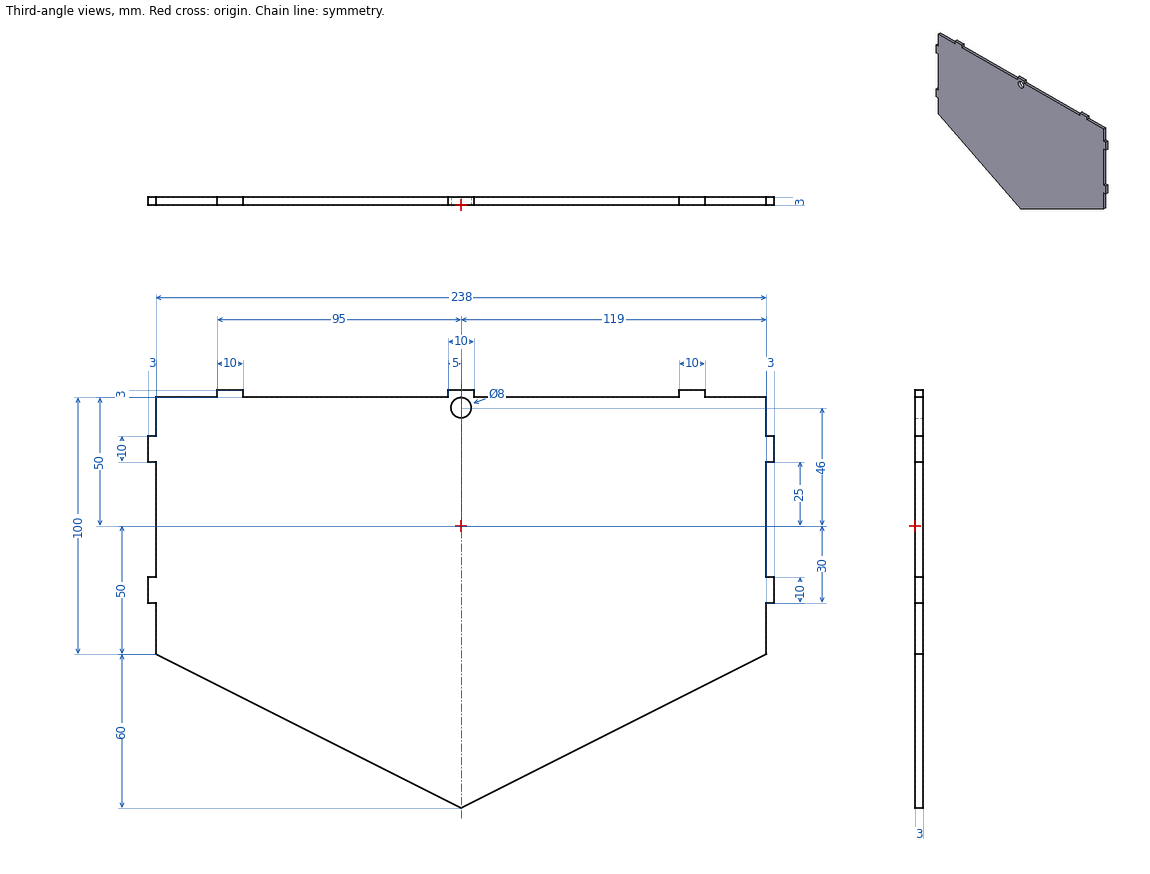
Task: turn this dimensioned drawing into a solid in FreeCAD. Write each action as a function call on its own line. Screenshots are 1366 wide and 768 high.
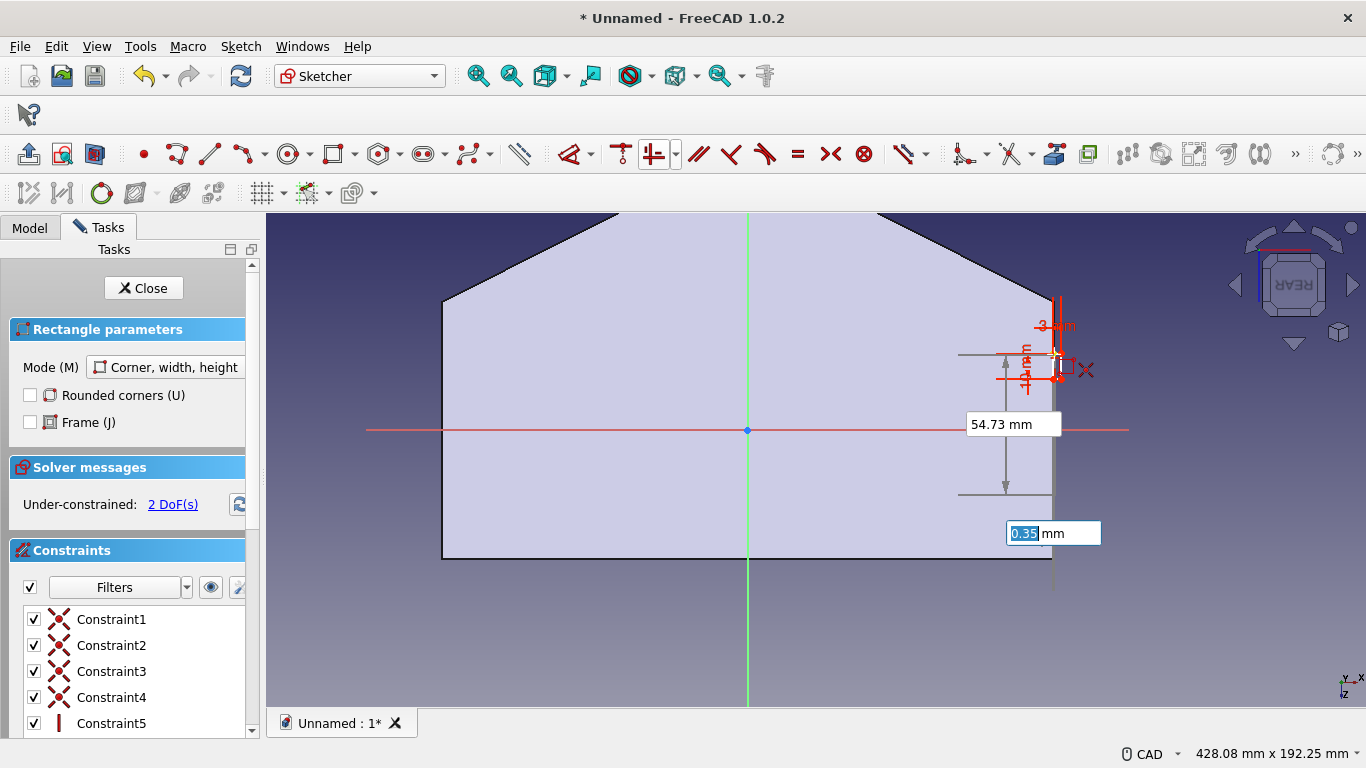
click(1061, 520)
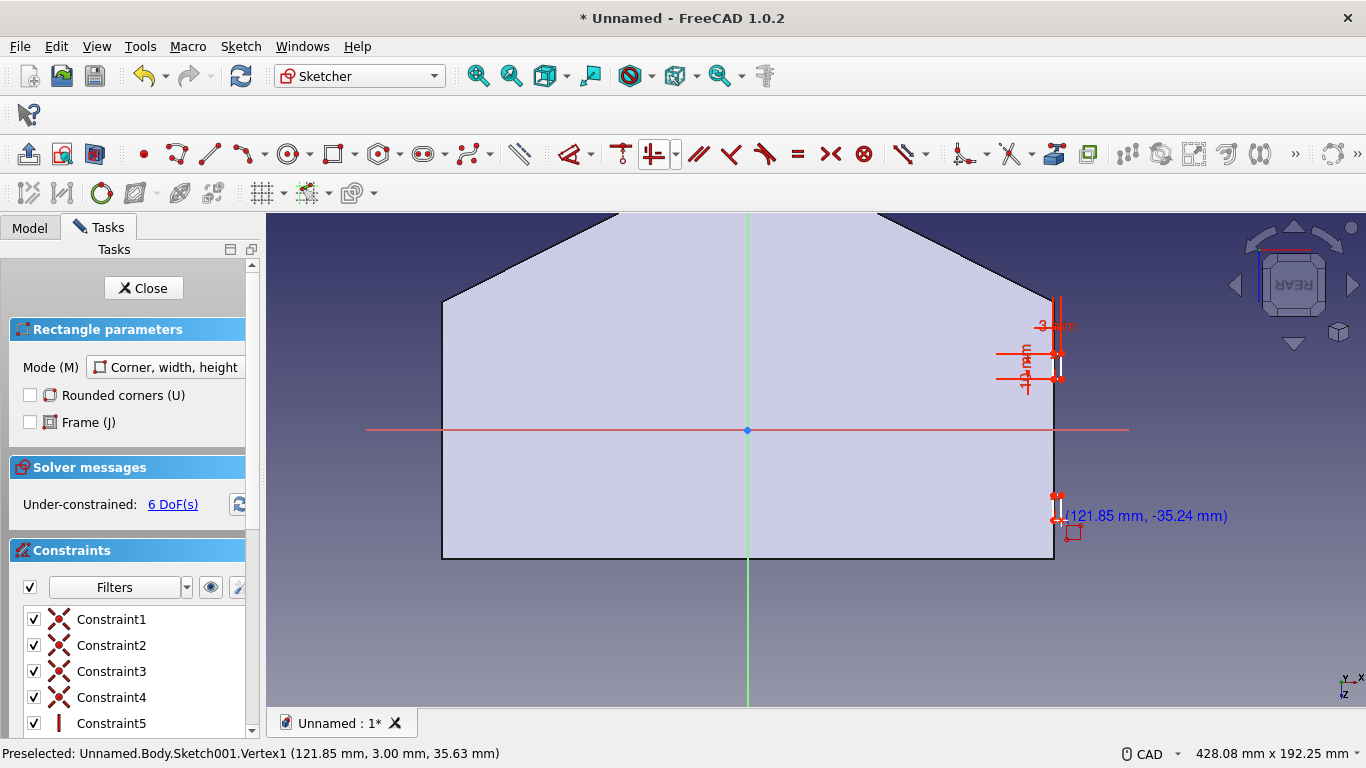
scroll(434, 495, up, 4)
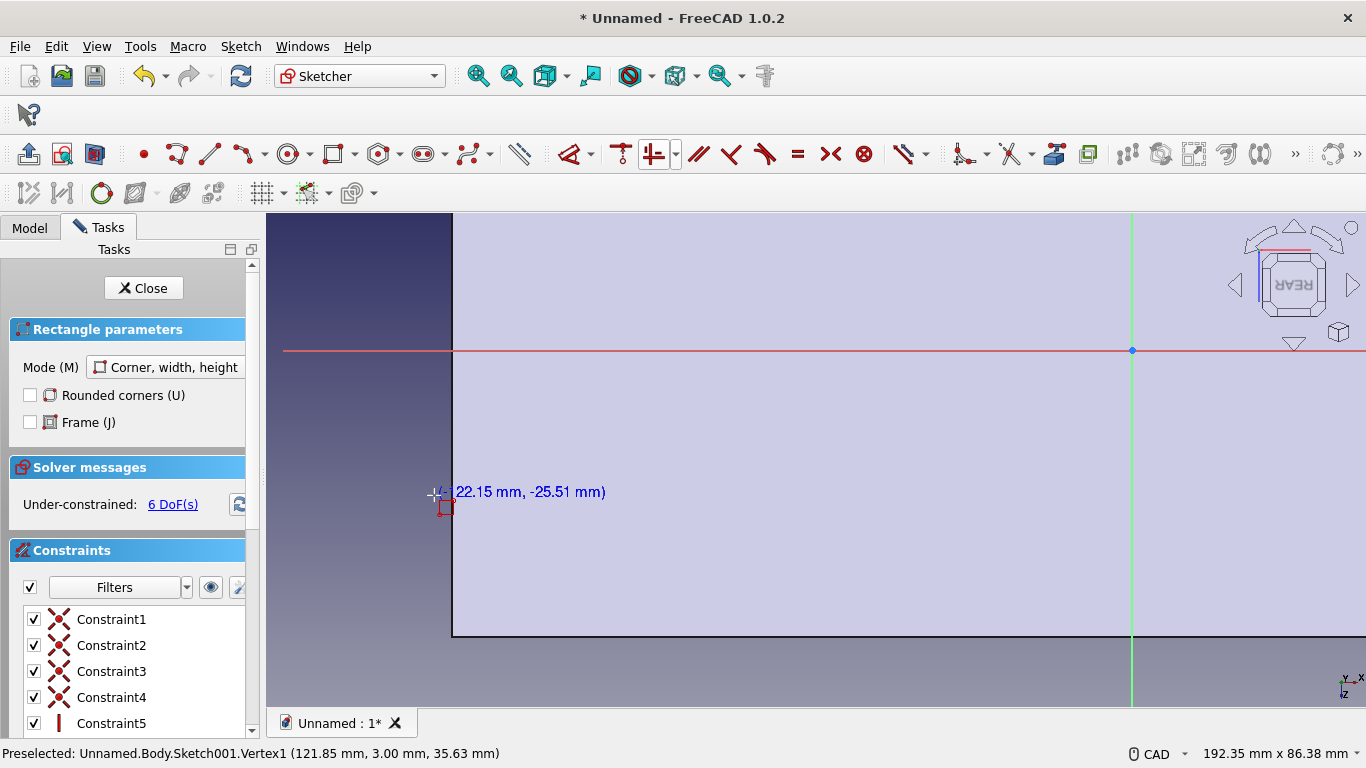
click(435, 494)
move(452, 551)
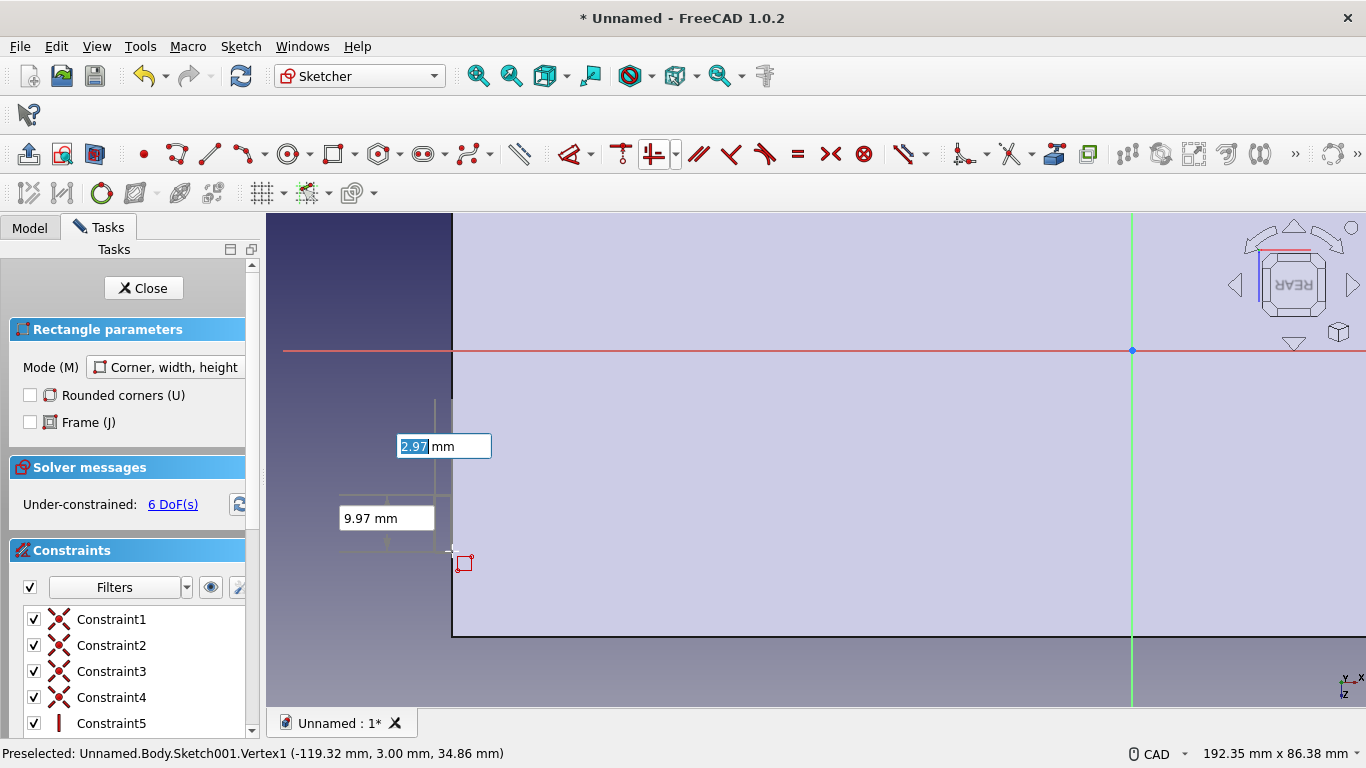
text(3)
key(Tab)
text(10)
key(Return)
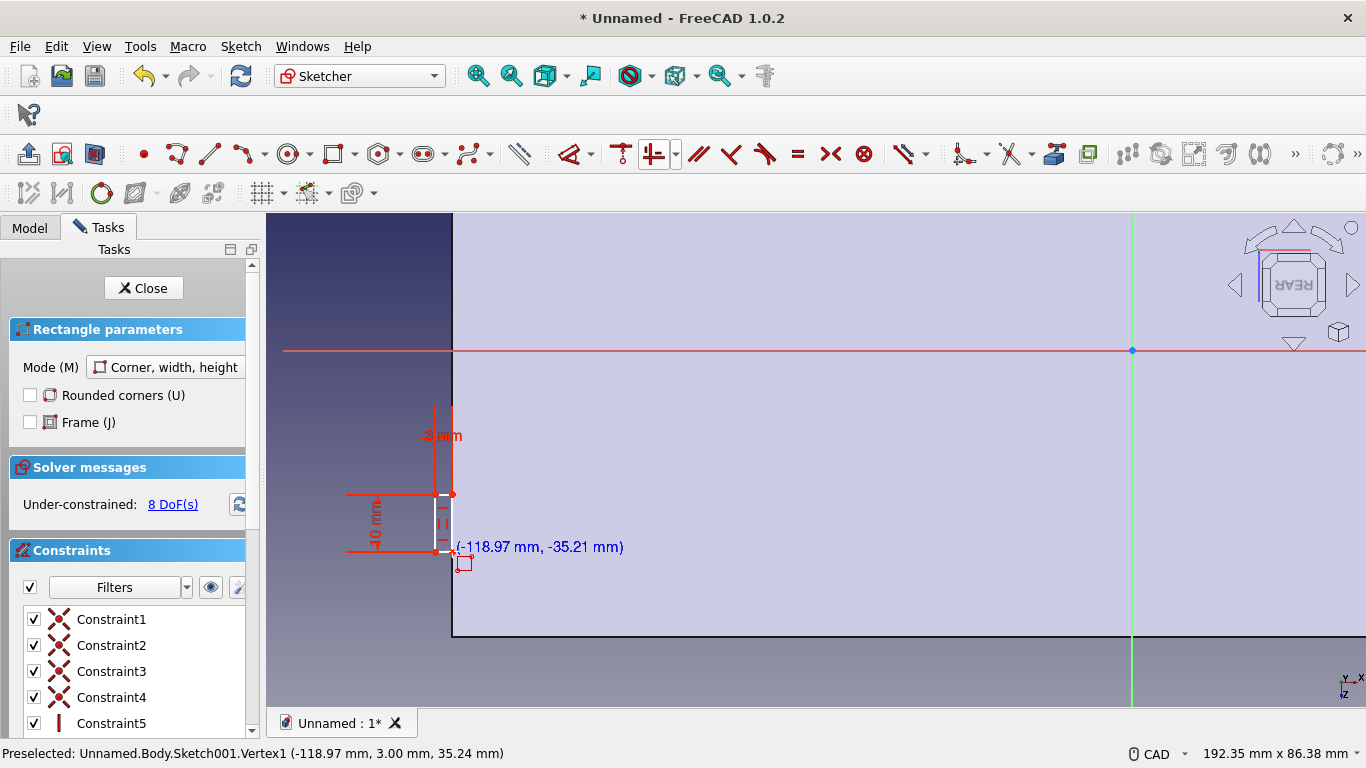
scroll(433, 496, down, 4)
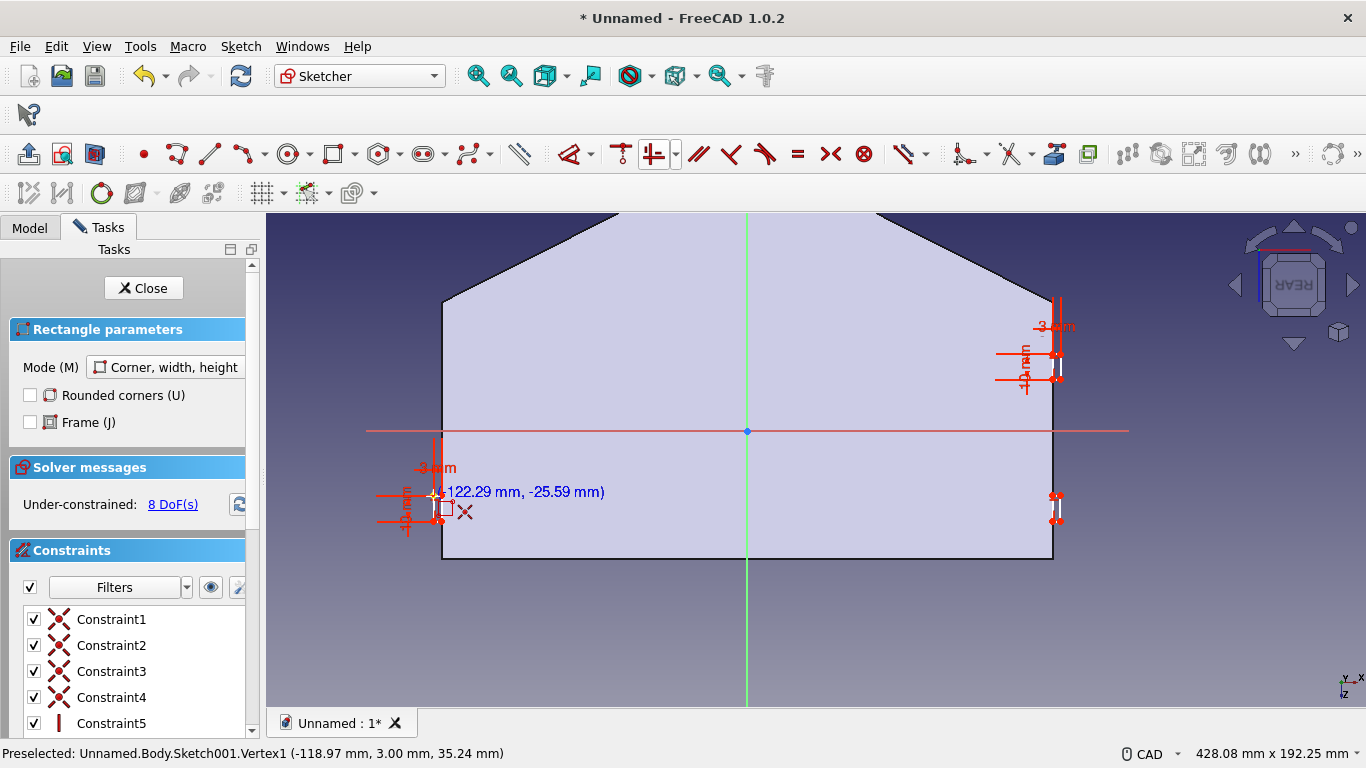
scroll(434, 354, up, 4)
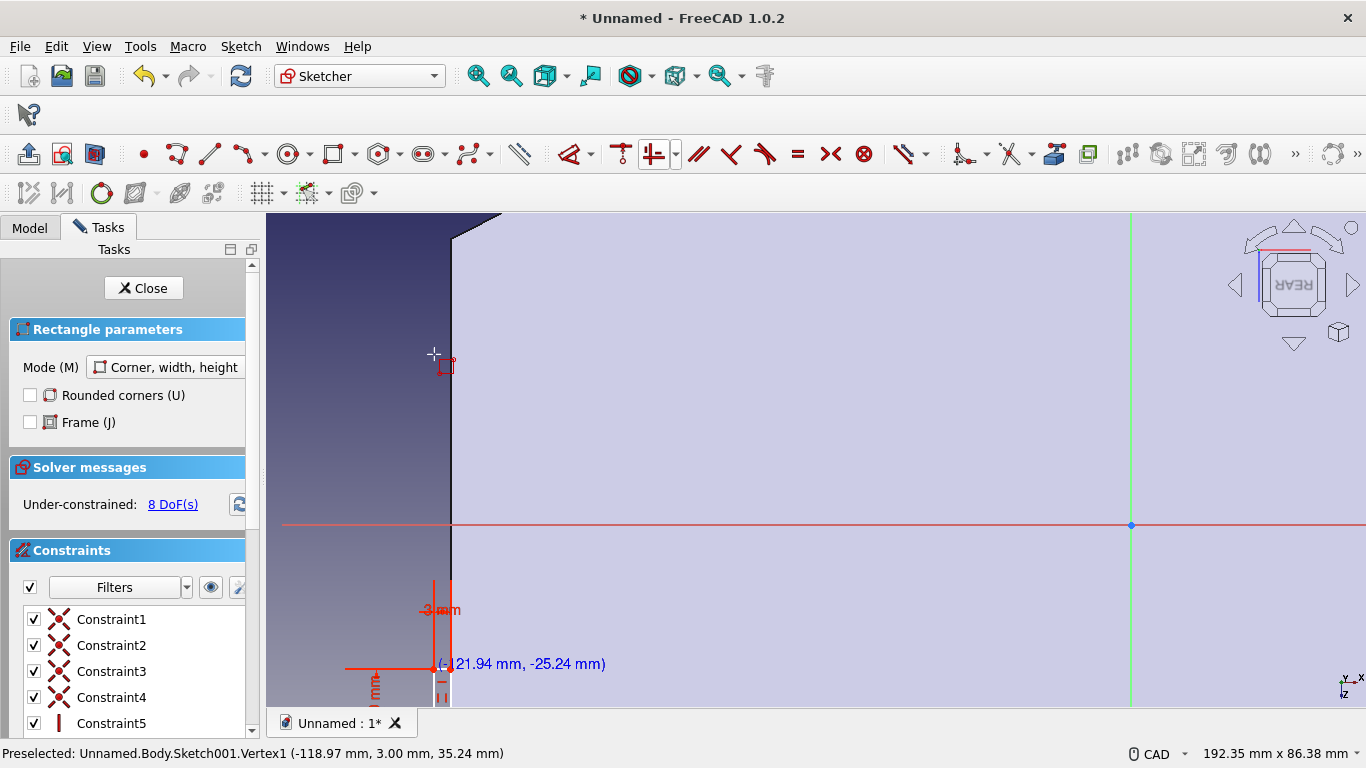
click(433, 353)
move(451, 411)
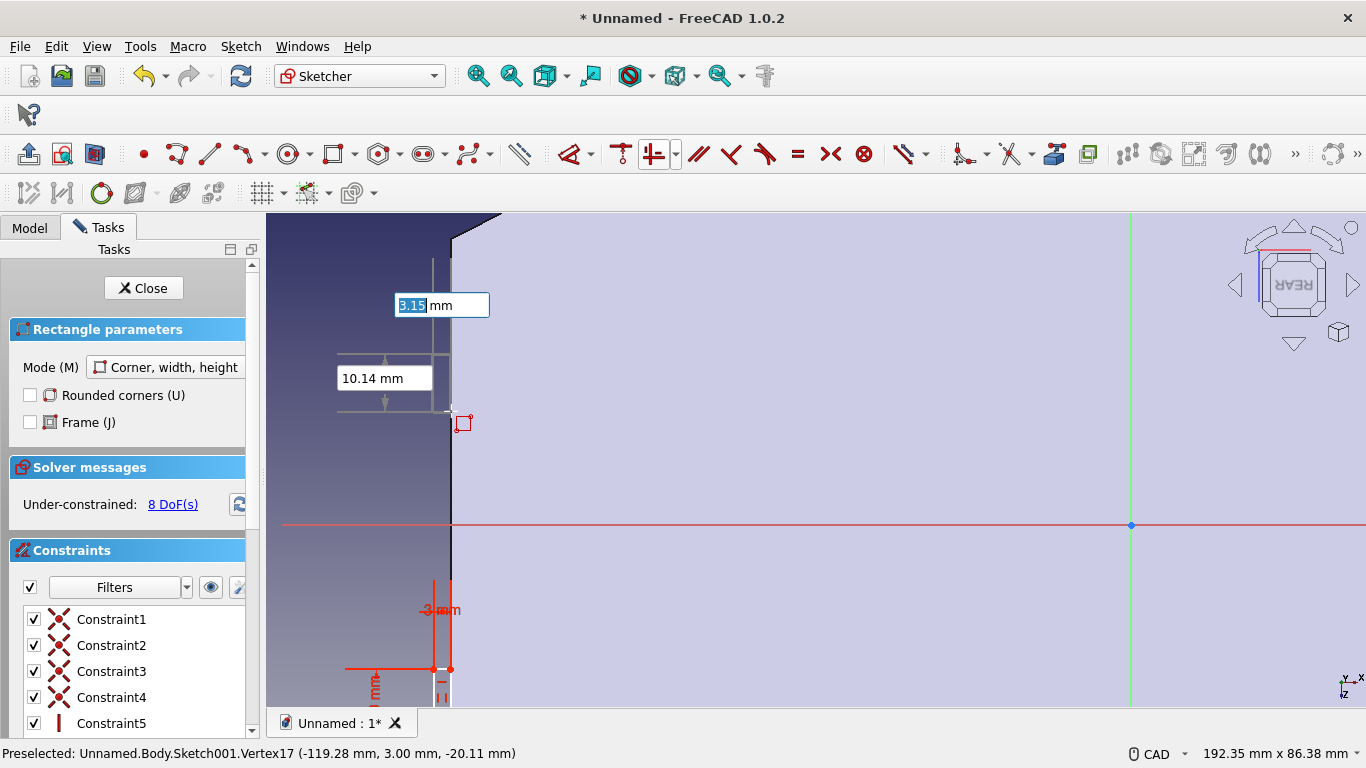
text(3)
key(Tab)
text(10)
key(Return)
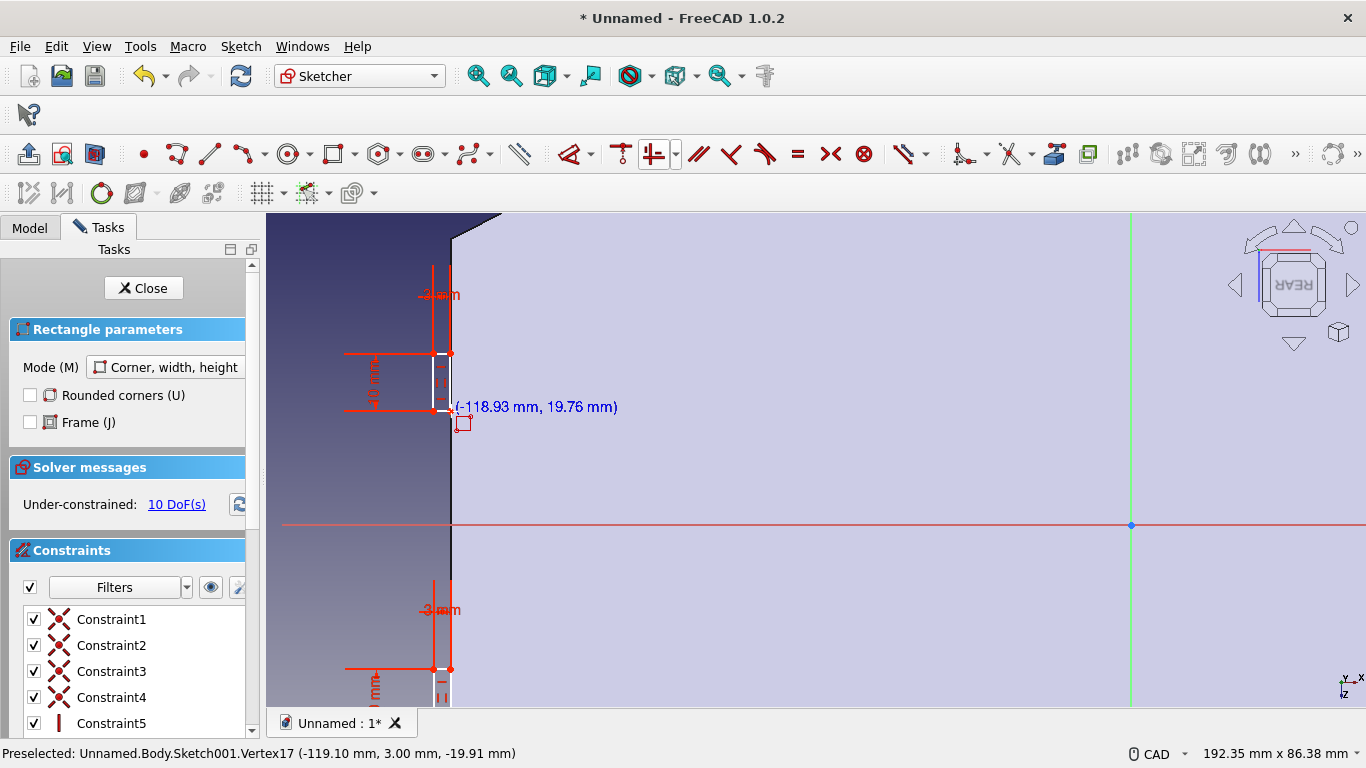
scroll(434, 353, down, 4)